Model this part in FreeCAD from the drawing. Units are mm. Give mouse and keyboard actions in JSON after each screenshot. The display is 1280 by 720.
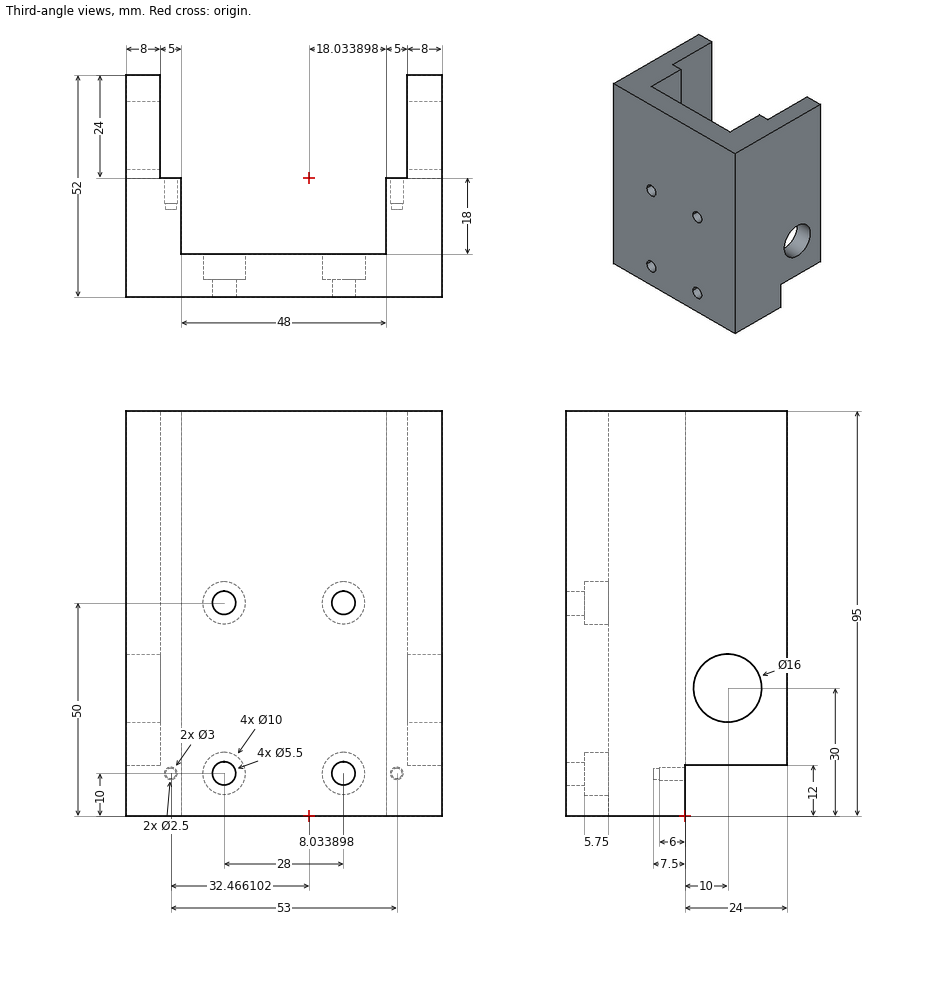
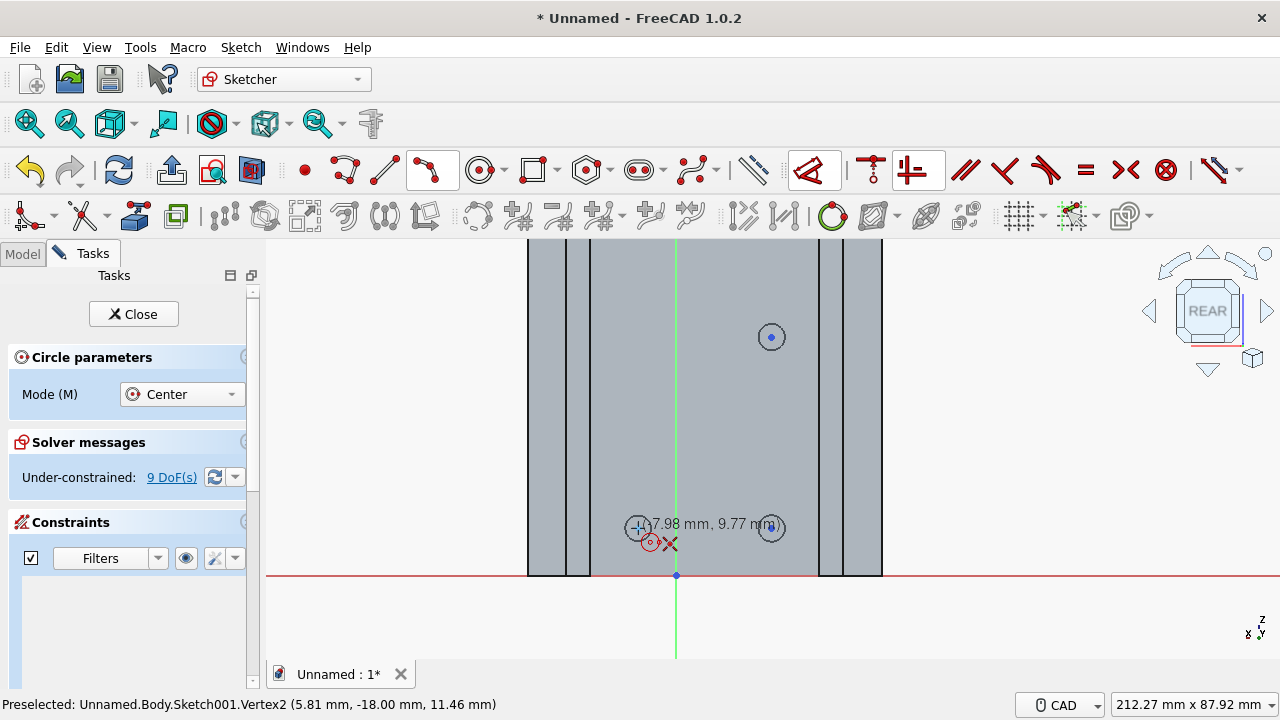
{"action": "scroll", "coordinate": [638, 337], "scroll_direction": "up", "scroll_amount": 3}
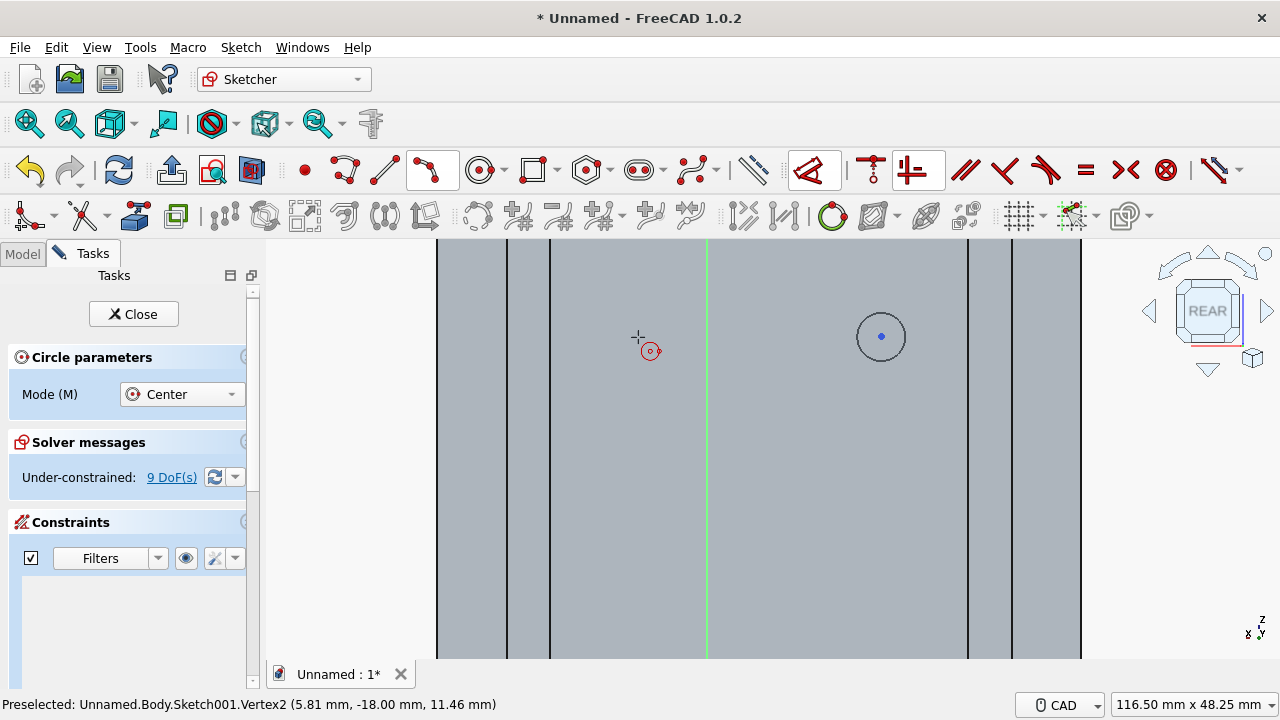
{"action": "left_click", "coordinate": [638, 336]}
{"action": "left_click", "coordinate": [654, 319]}
{"action": "key", "text": "Escape"}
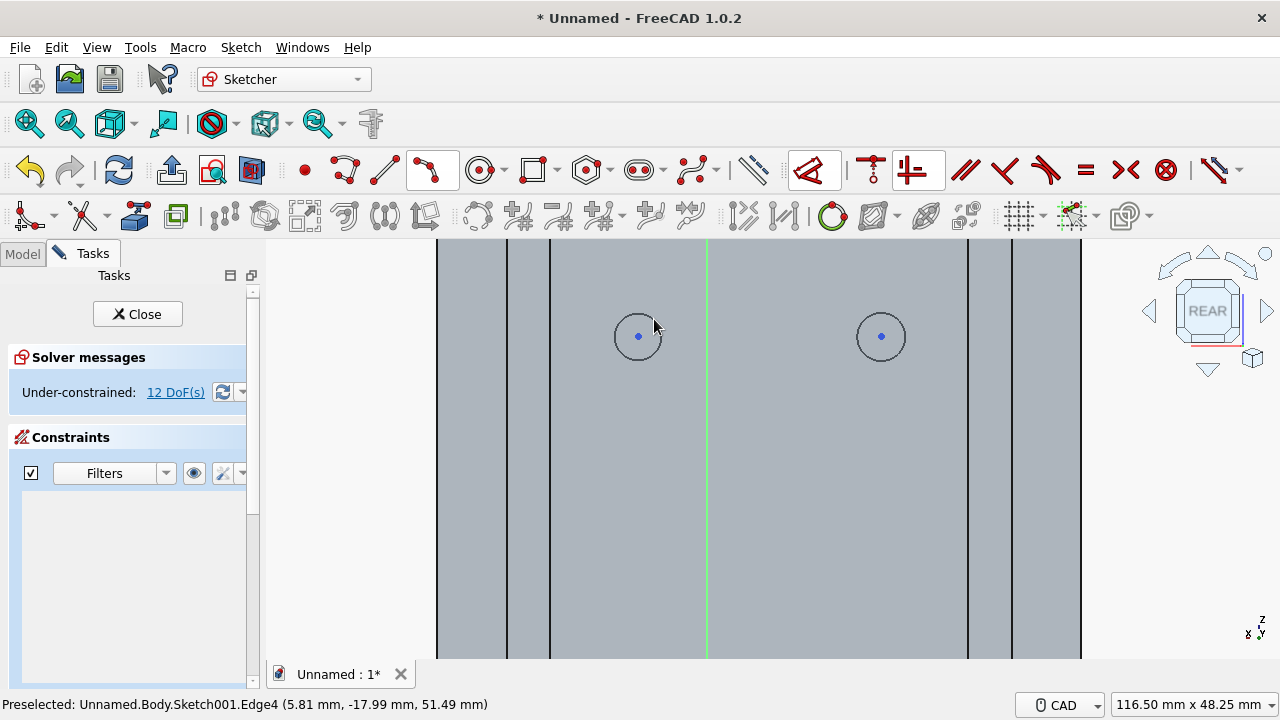
{"action": "scroll", "coordinate": [638, 336], "scroll_direction": "down", "scroll_amount": 3}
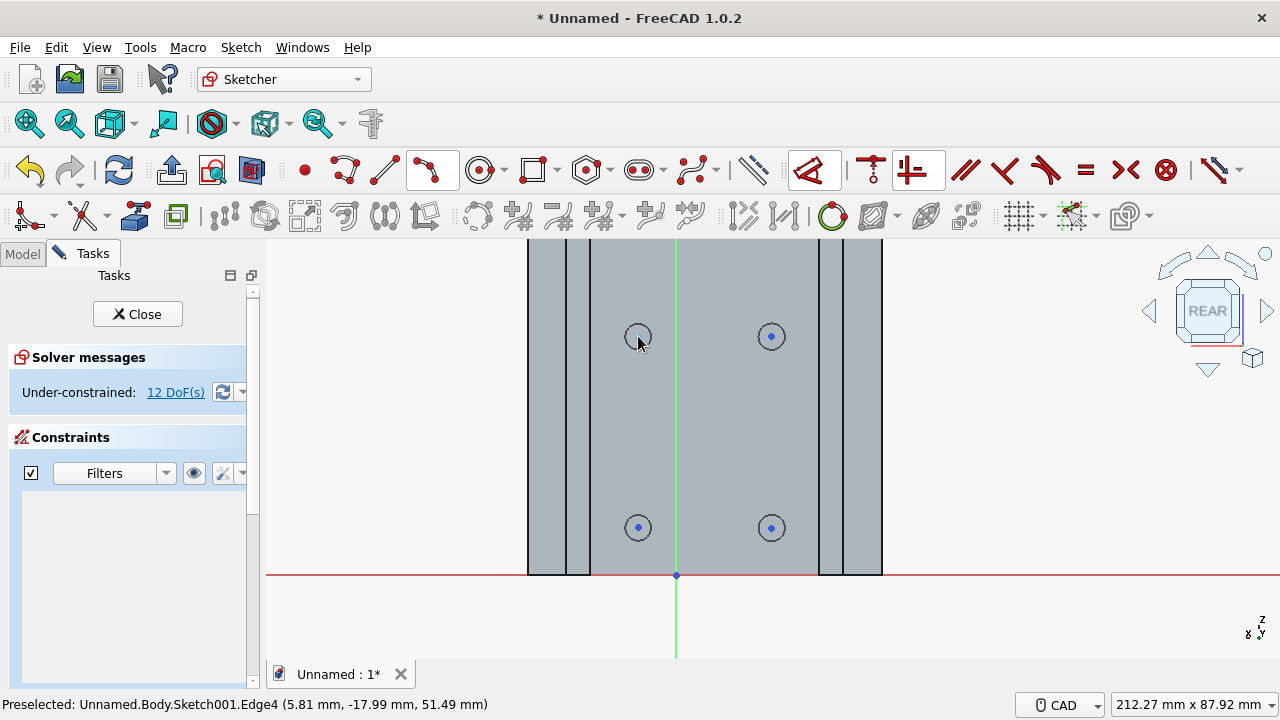
{"action": "left_click", "coordinate": [781, 519]}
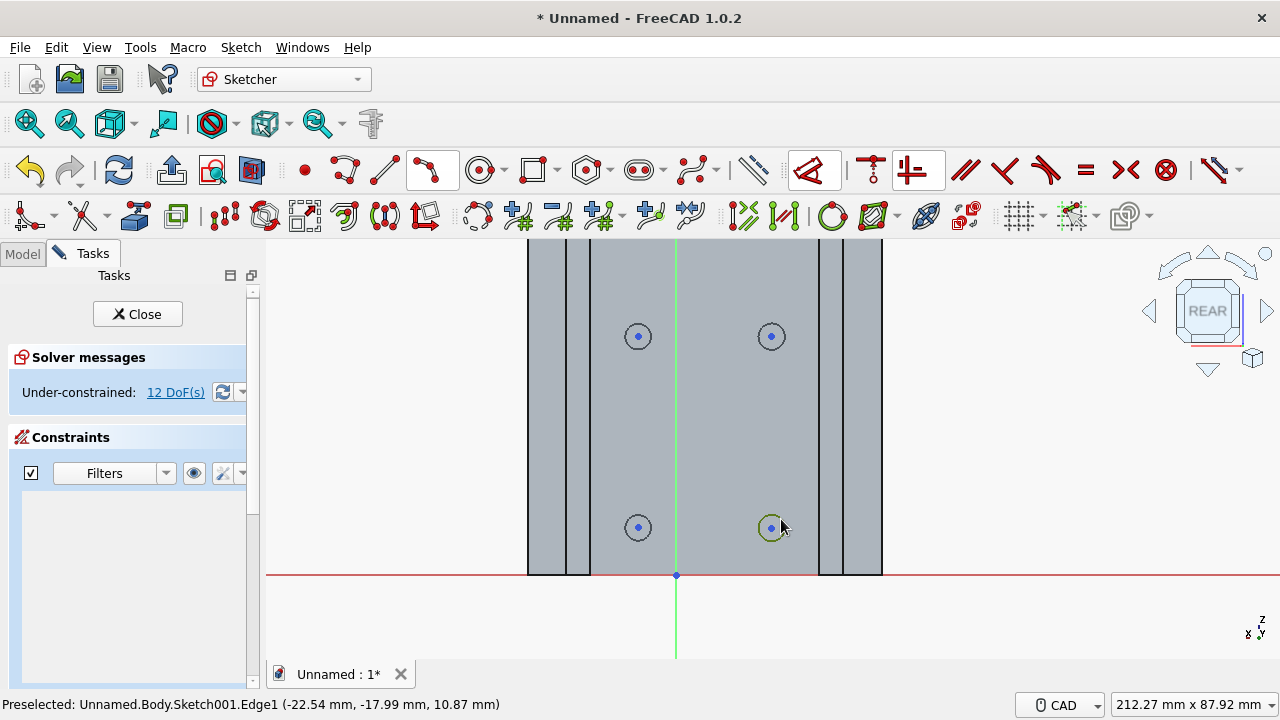
{"action": "left_click", "coordinate": [781, 327]}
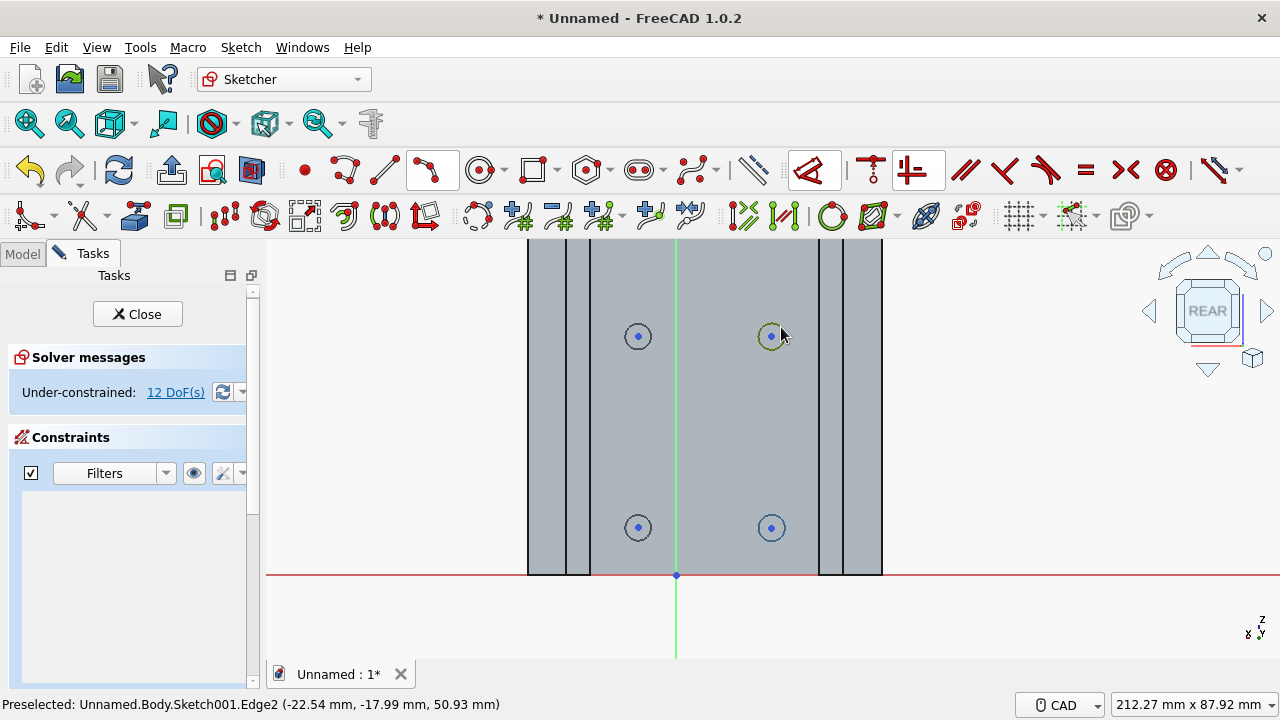
{"action": "left_click", "coordinate": [647, 519]}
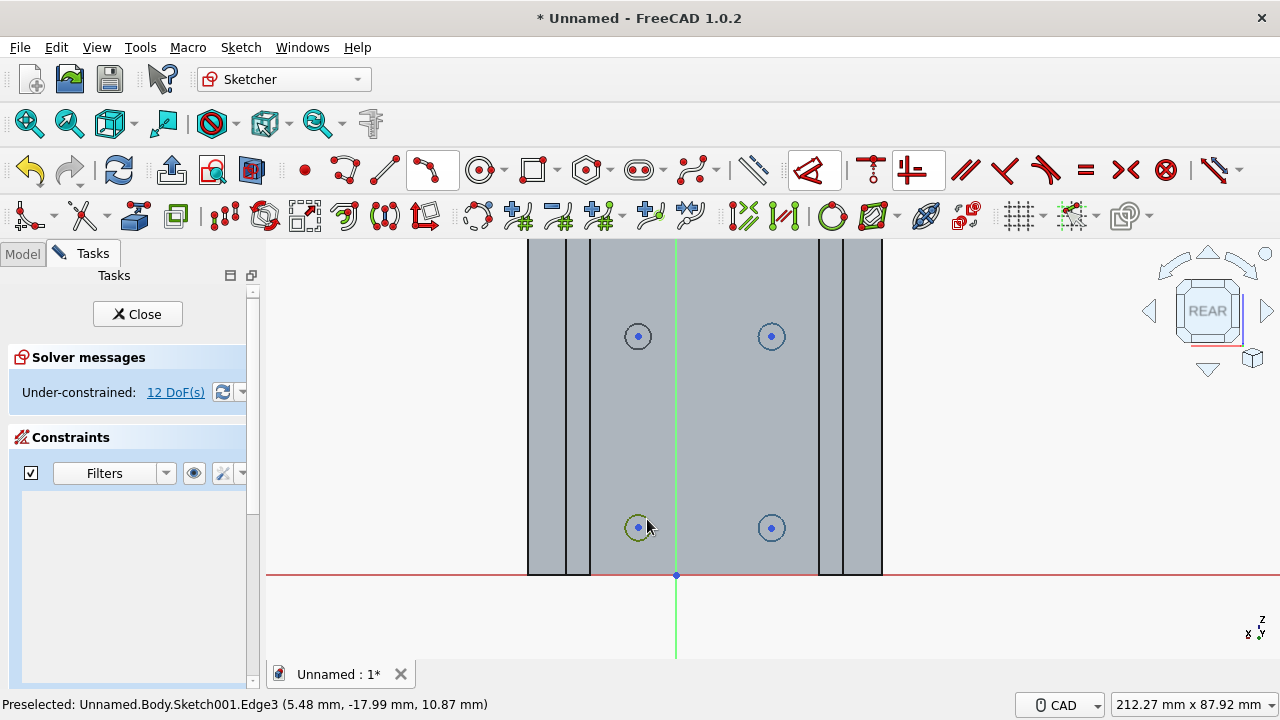
{"action": "left_click", "coordinate": [647, 328]}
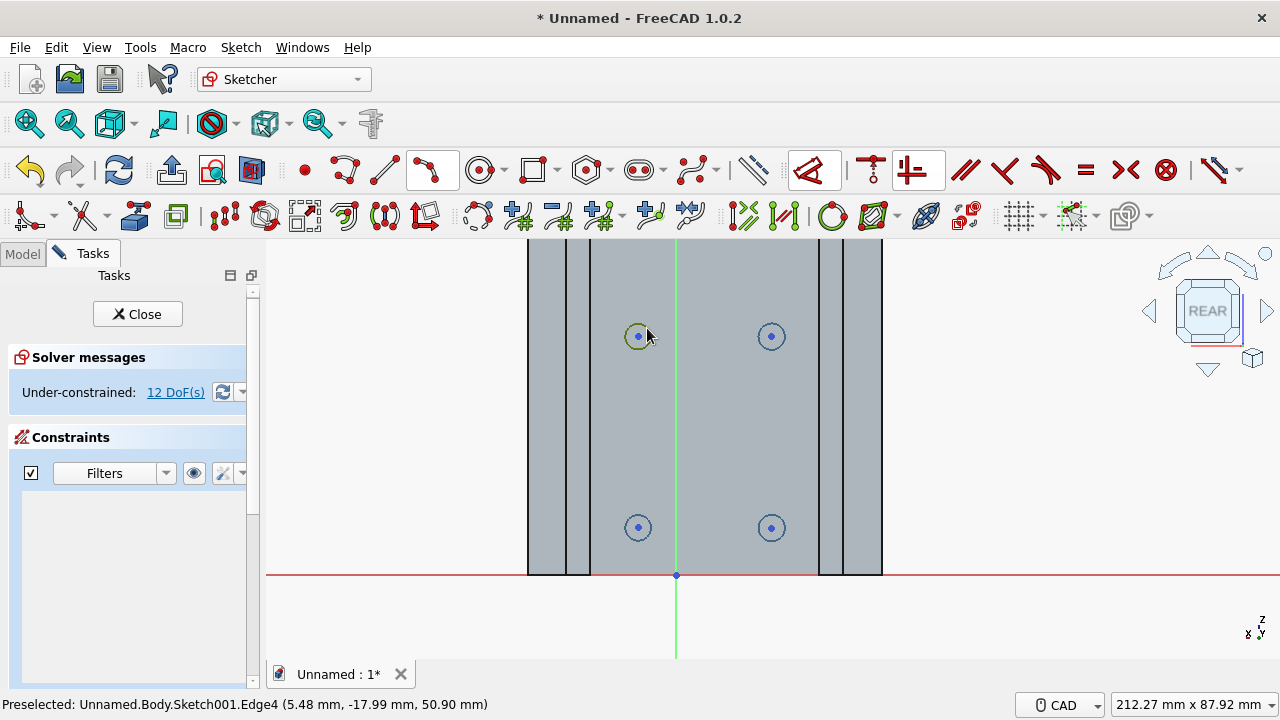
{"action": "left_click", "coordinate": [1086, 170]}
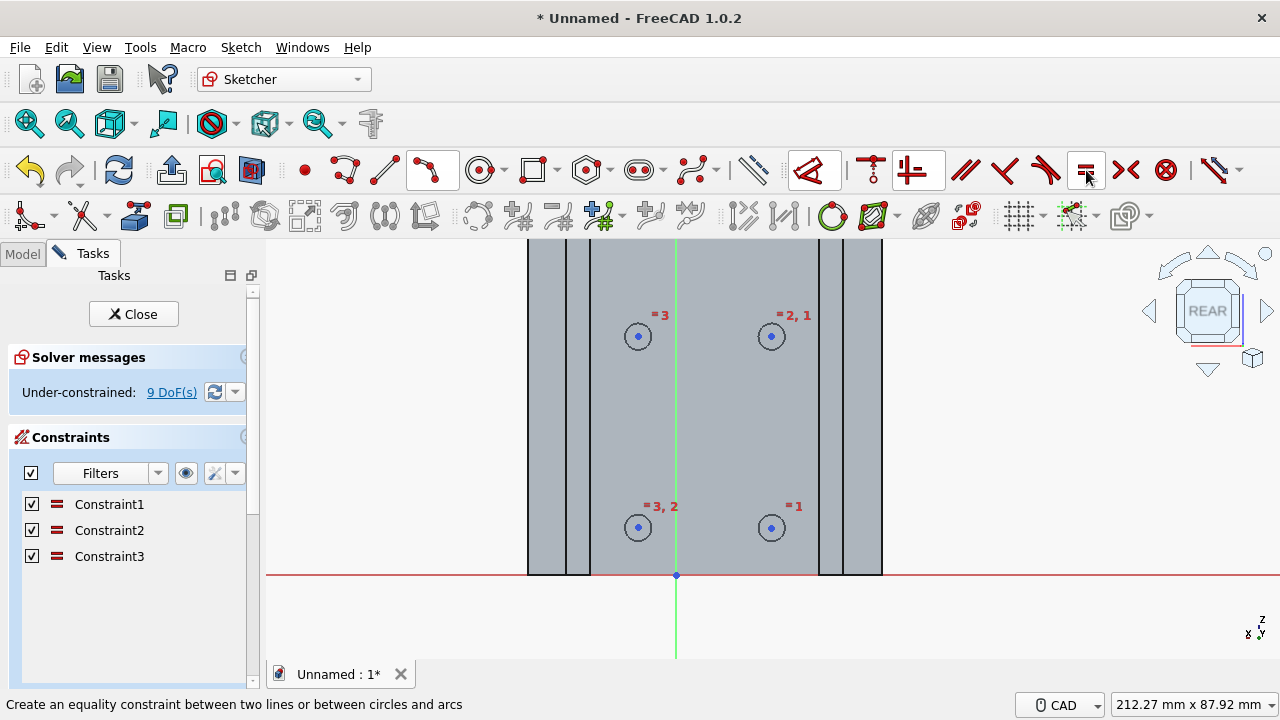
{"action": "left_click", "coordinate": [772, 528]}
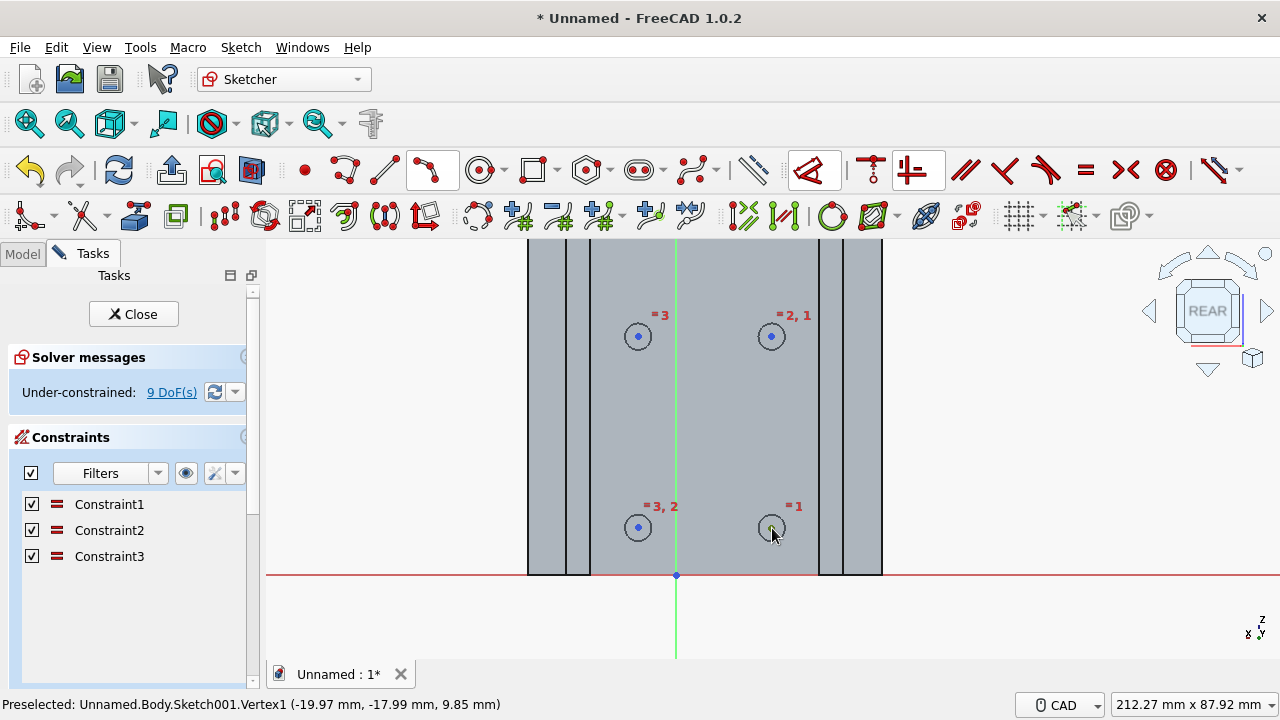
{"action": "left_click", "coordinate": [772, 337]}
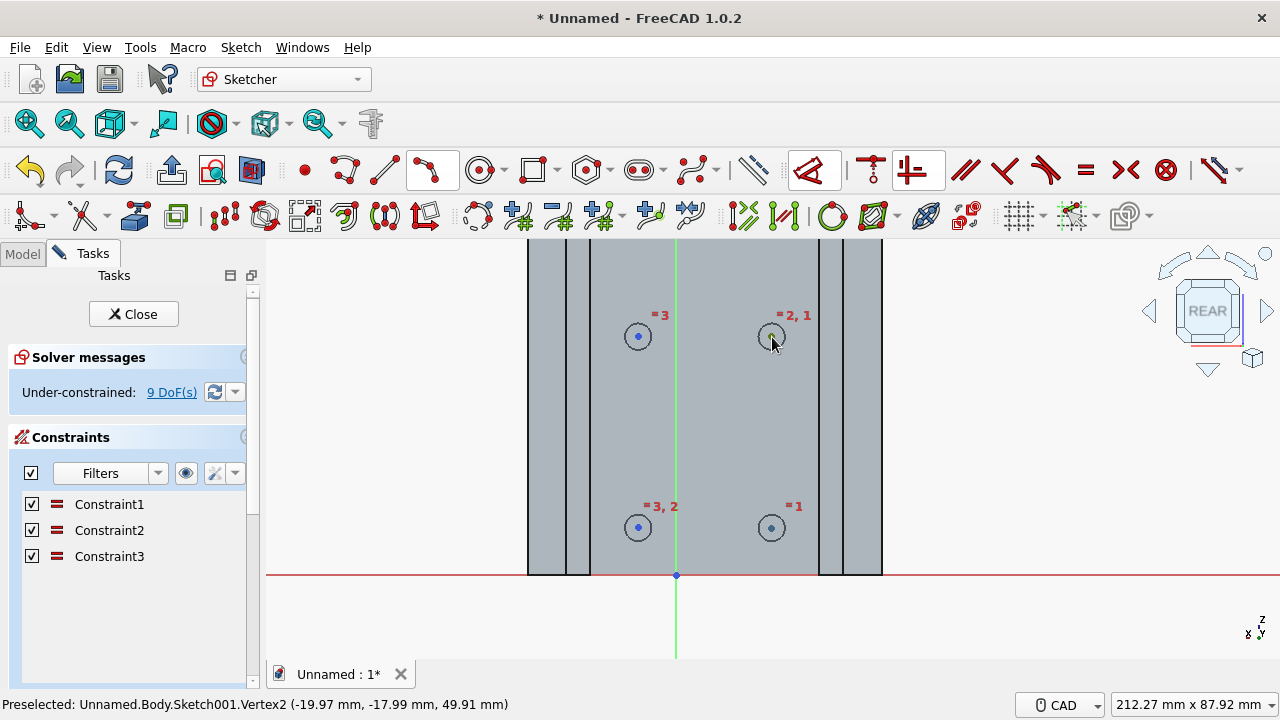
{"action": "left_click", "coordinate": [940, 170]}